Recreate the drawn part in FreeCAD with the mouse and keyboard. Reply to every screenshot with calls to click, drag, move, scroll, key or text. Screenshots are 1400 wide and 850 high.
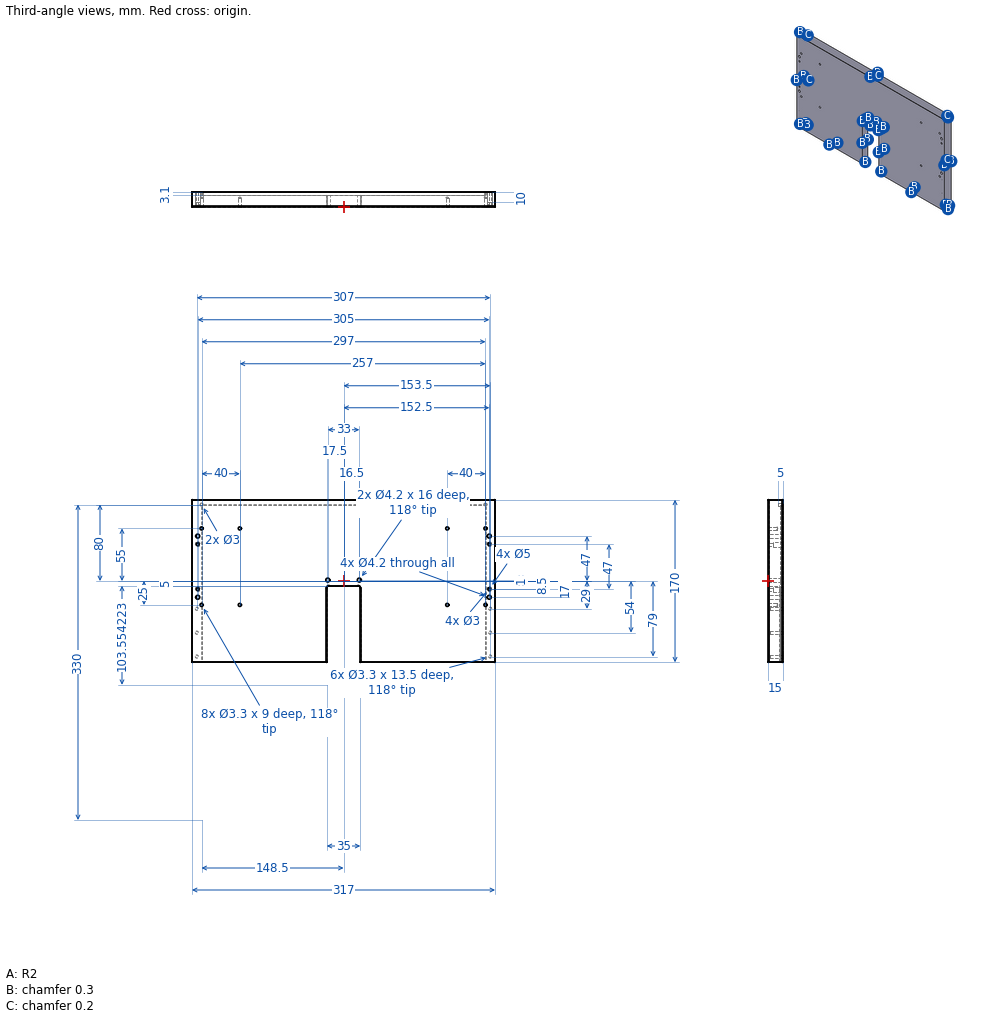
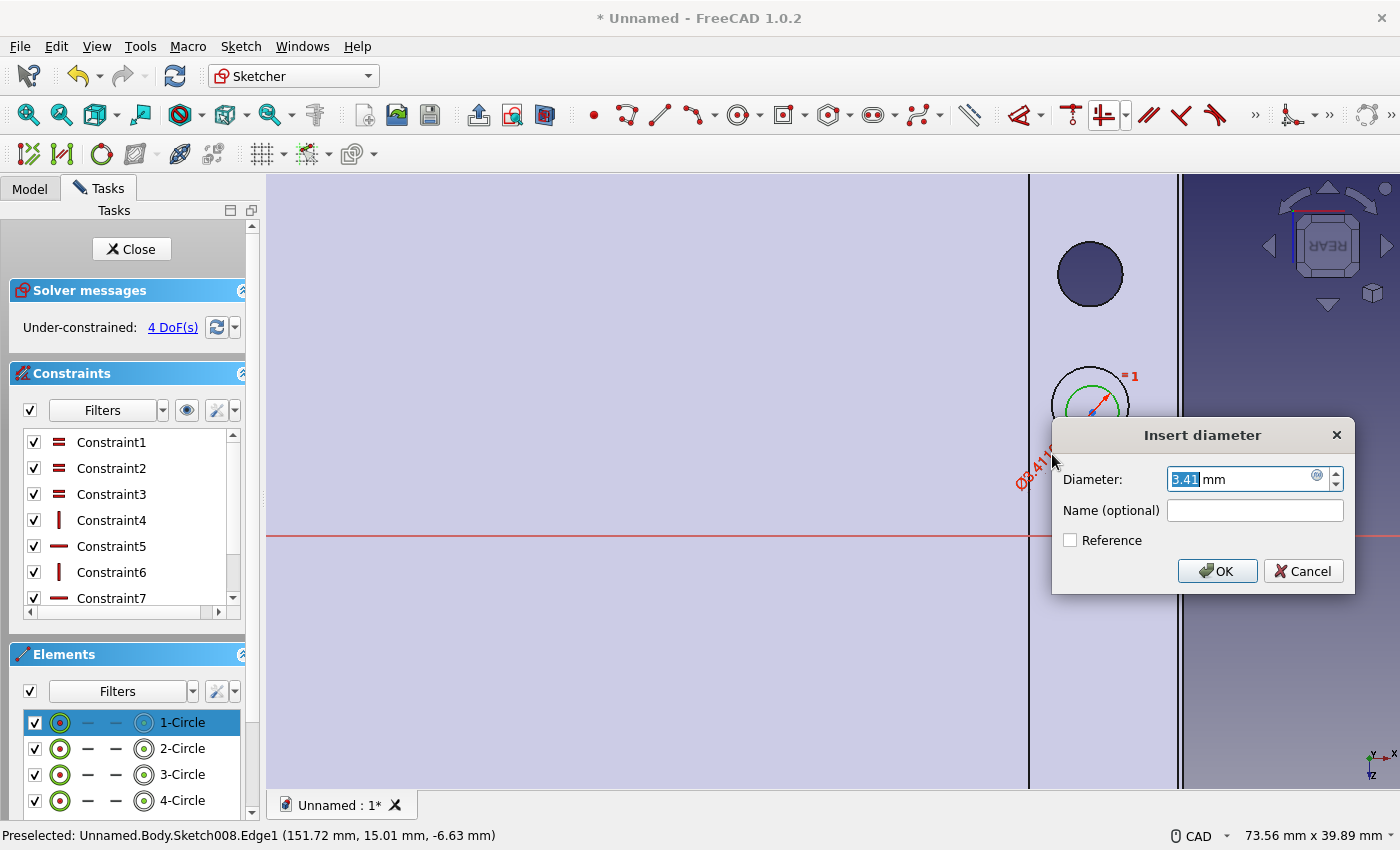
text(3)
key(Return)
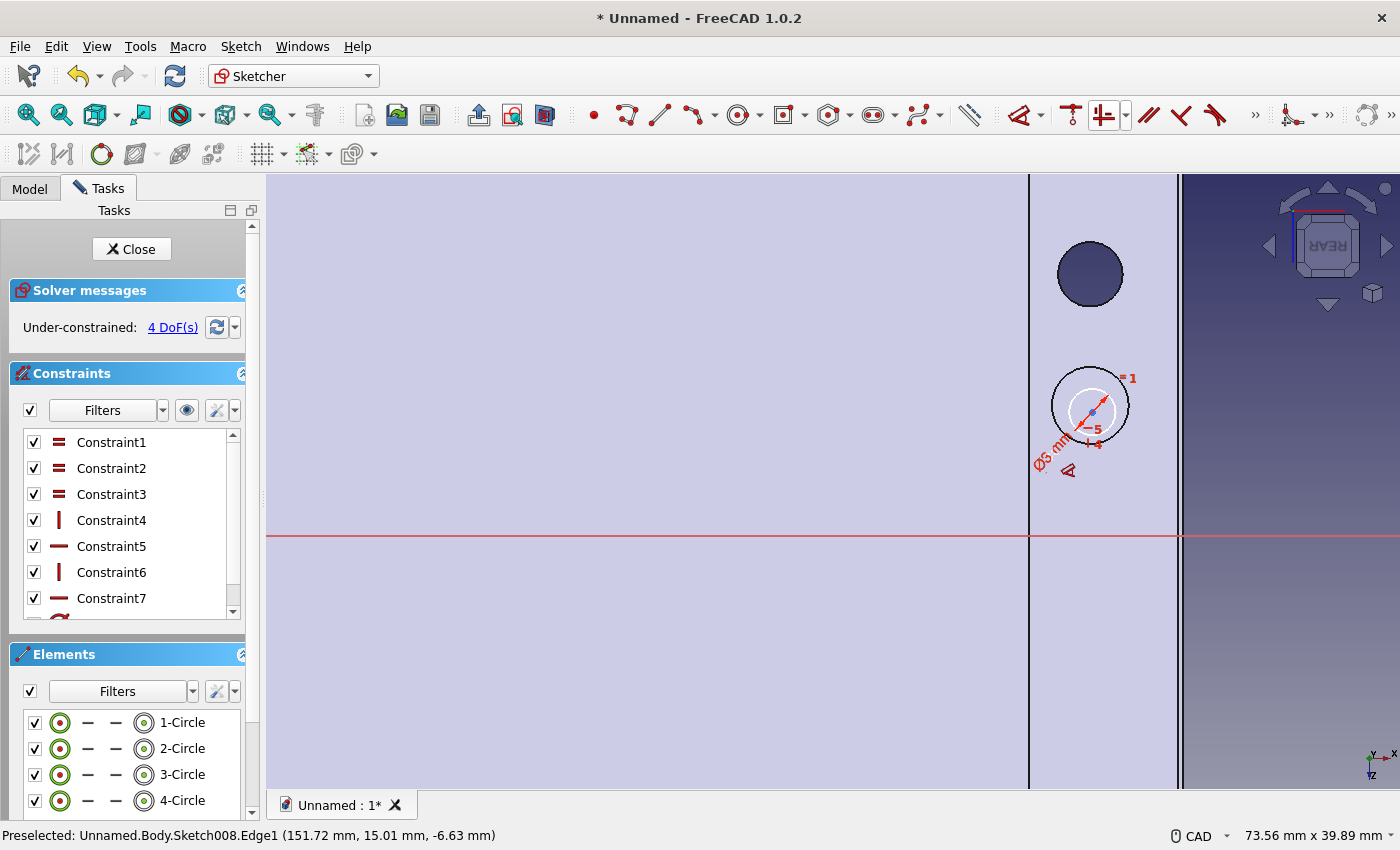
scroll(1081, 437, down, 10)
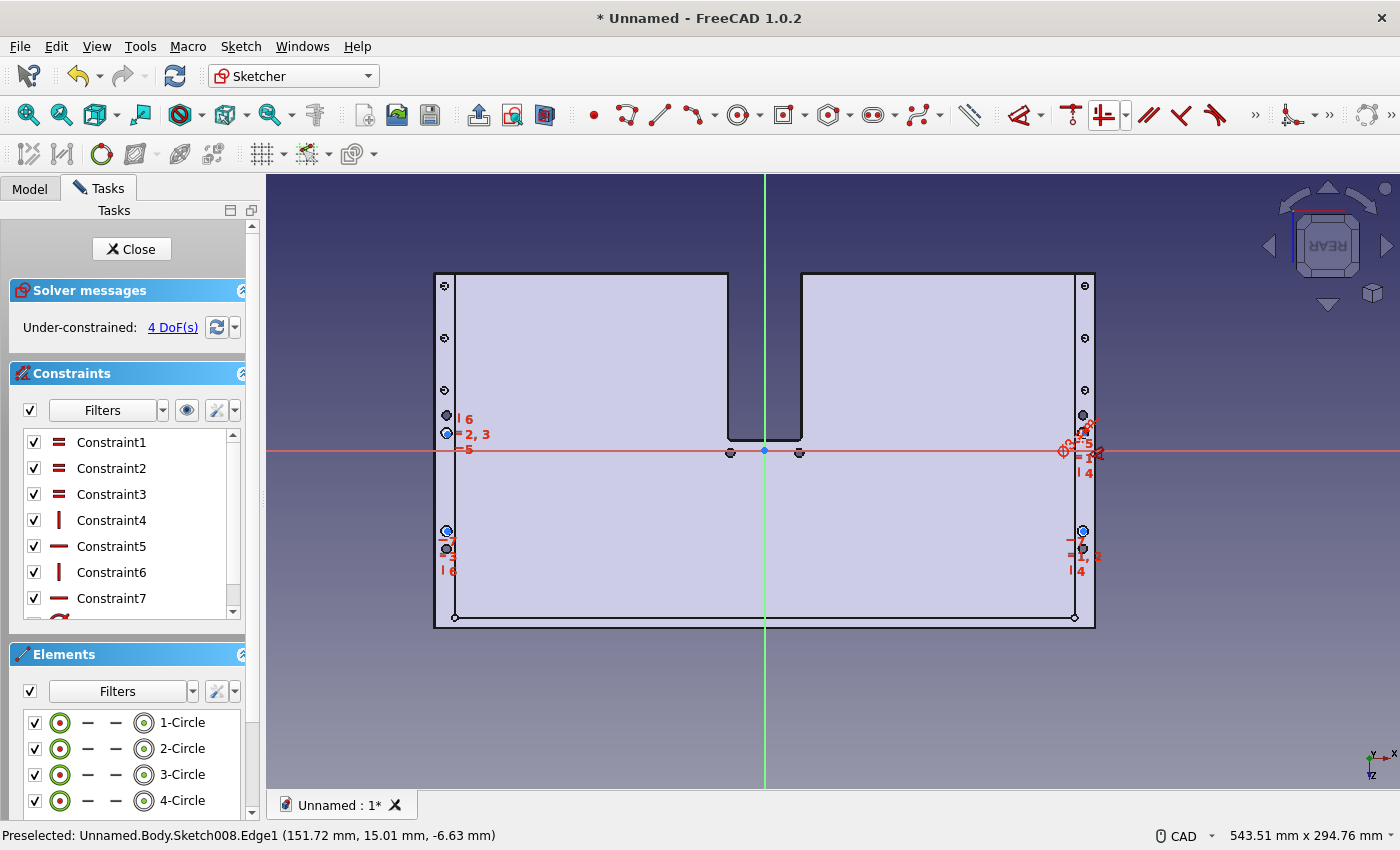
scroll(1083, 434, up, 5)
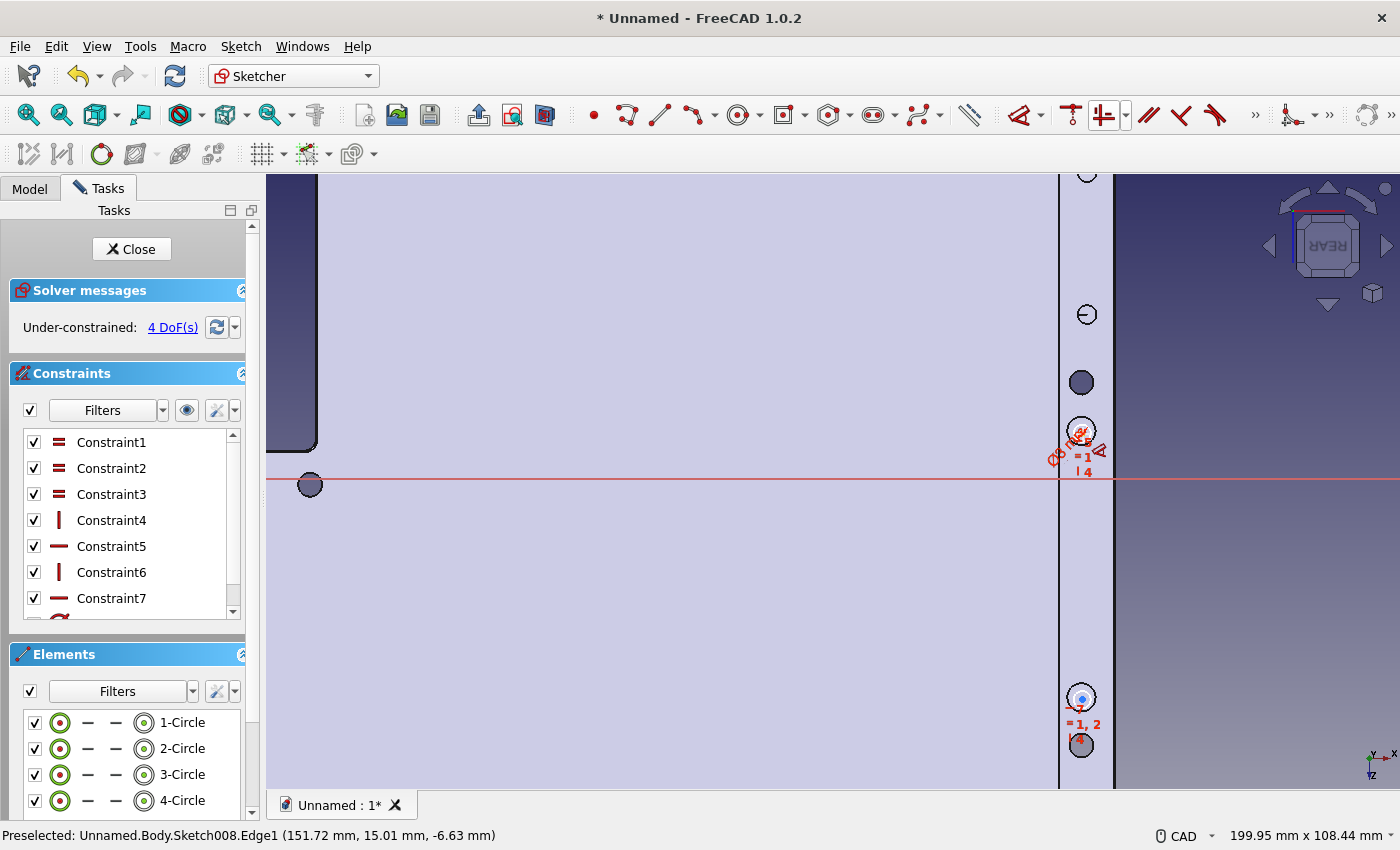
click(1082, 433)
click(1140, 456)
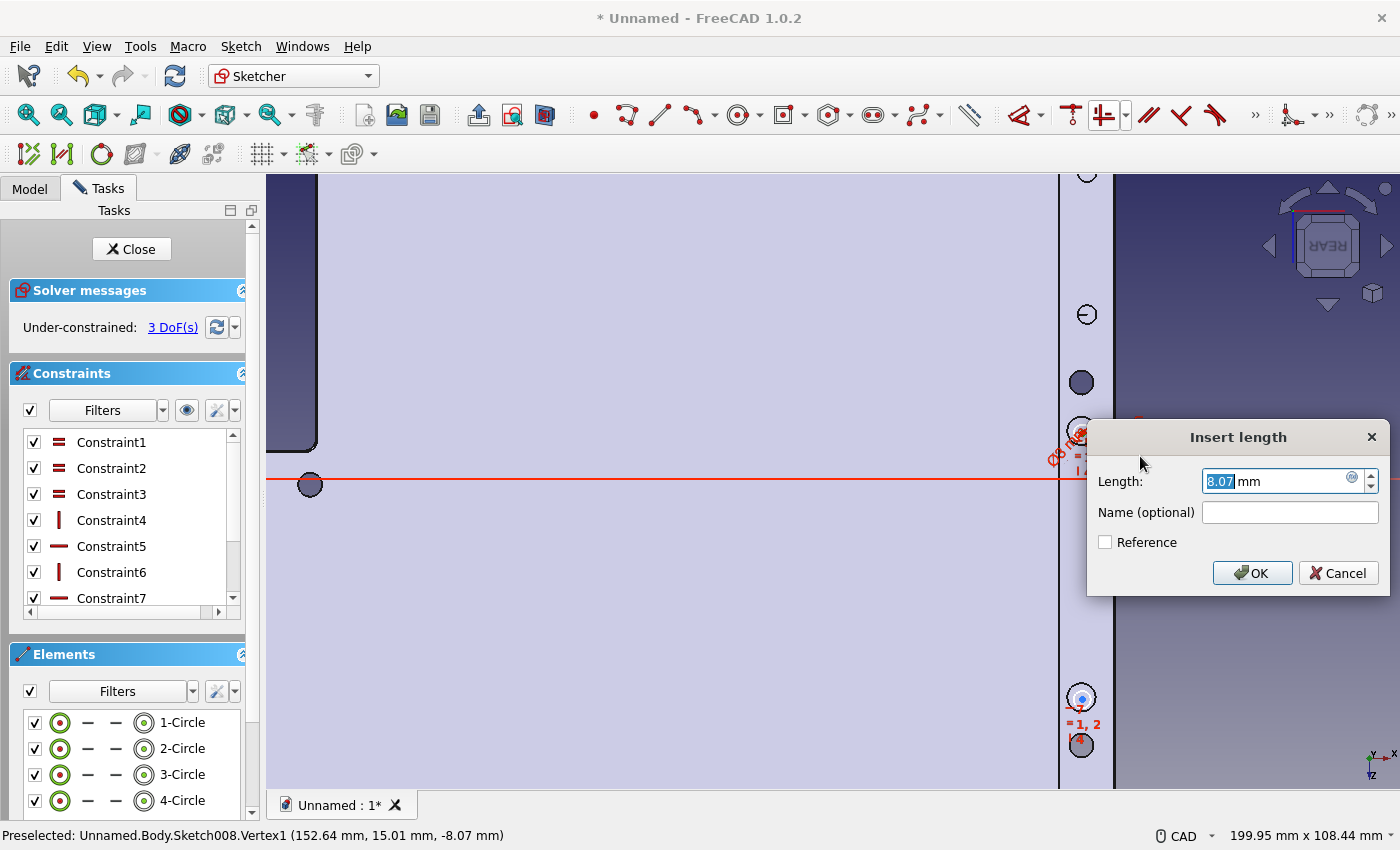
text(8.5)
key(Return)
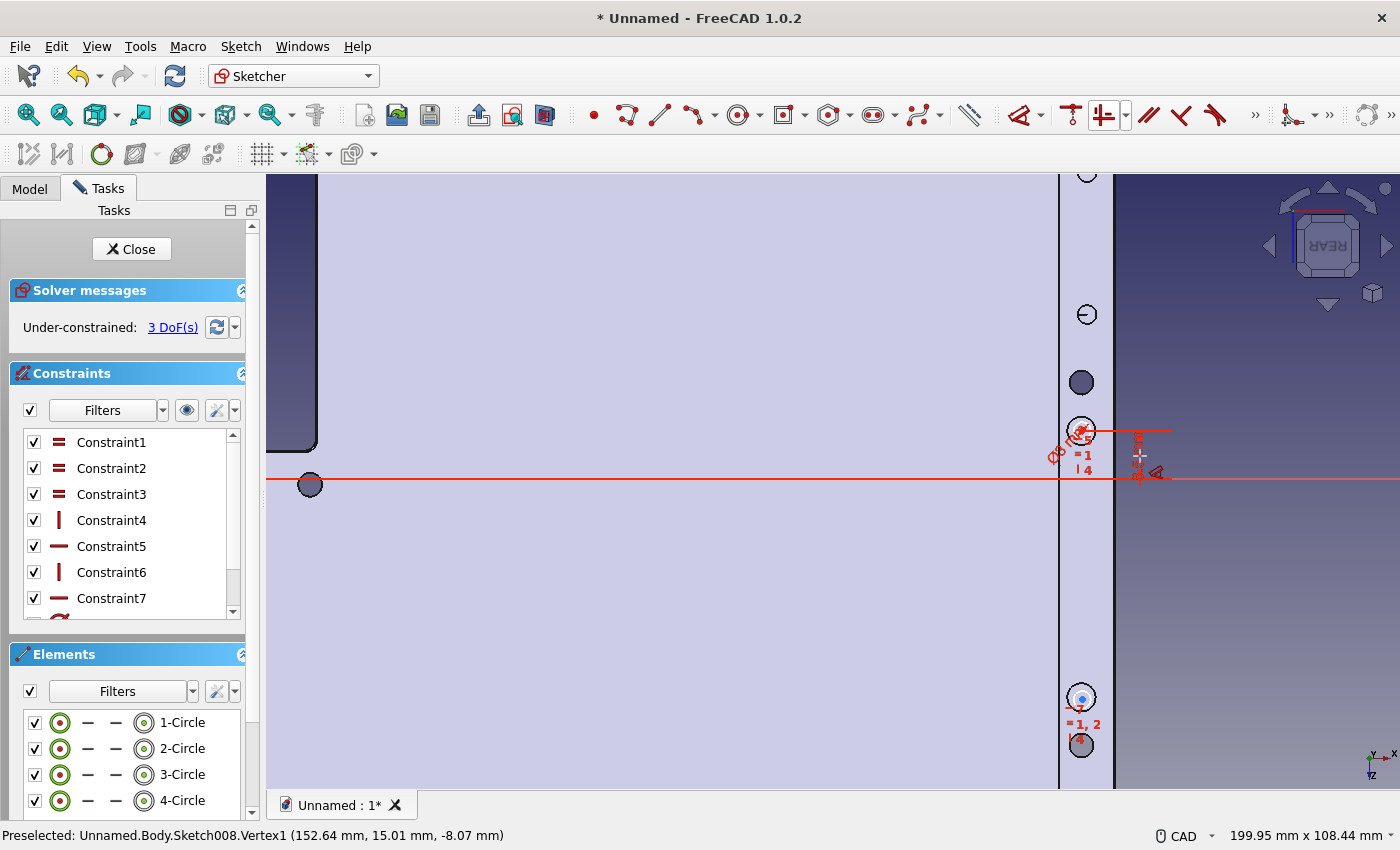
click(1082, 431)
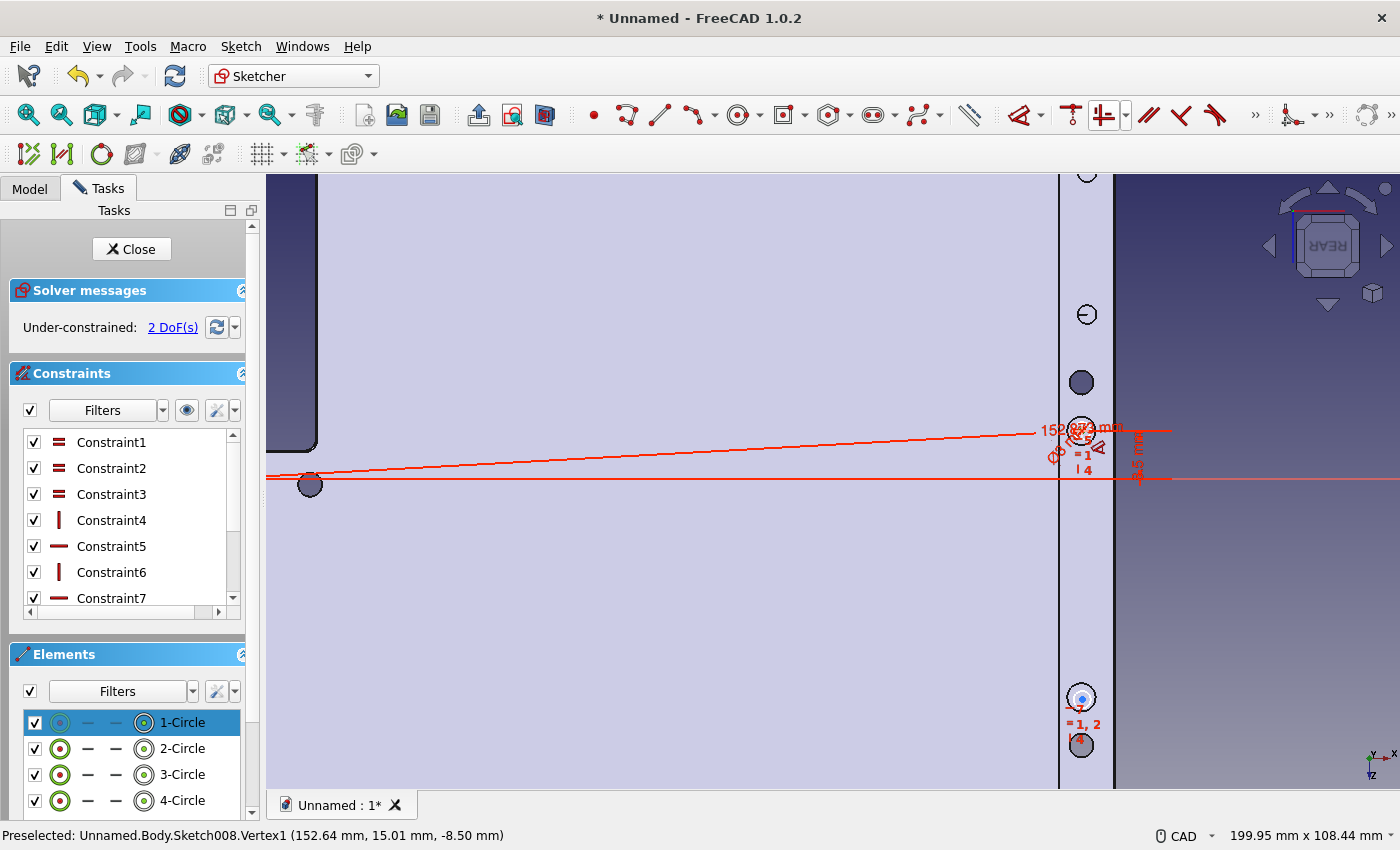
click(1082, 700)
click(1116, 565)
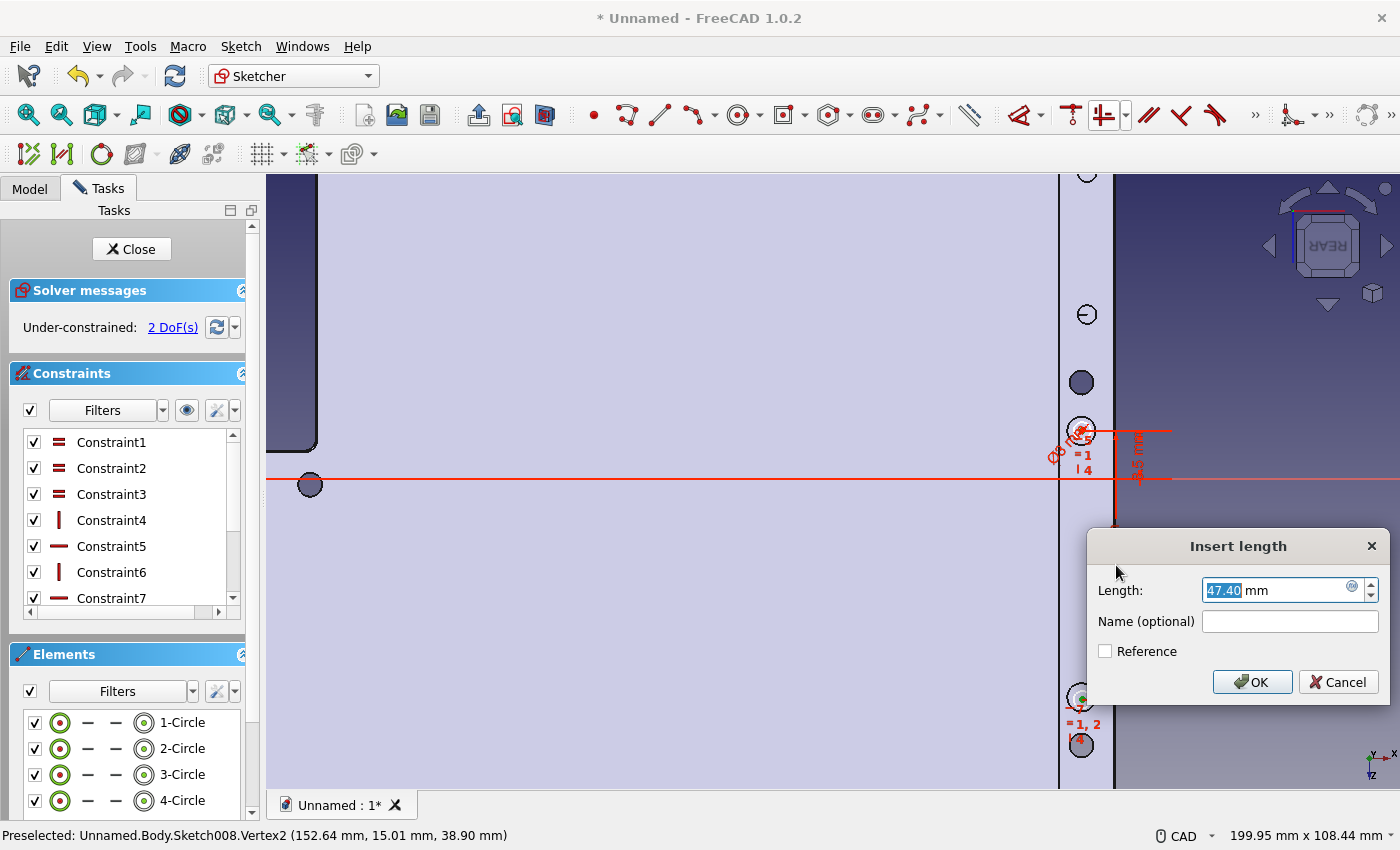
text(47)
key(Return)